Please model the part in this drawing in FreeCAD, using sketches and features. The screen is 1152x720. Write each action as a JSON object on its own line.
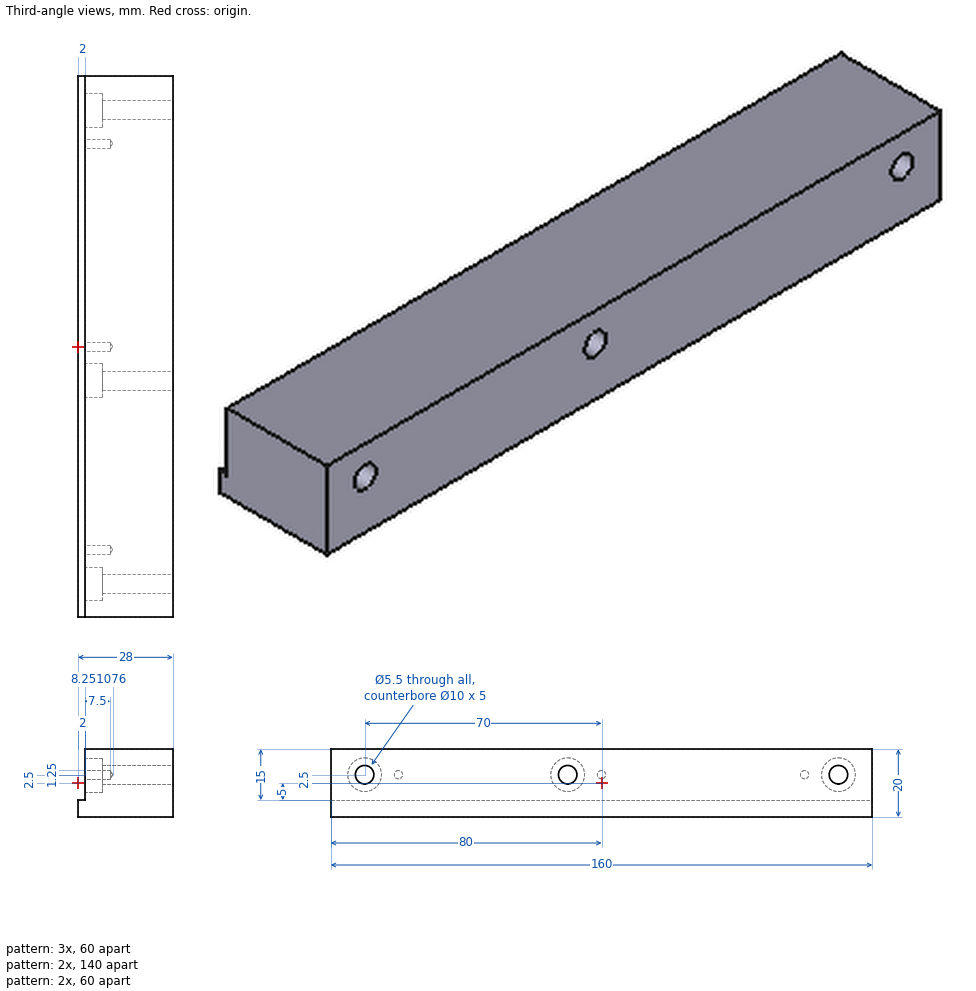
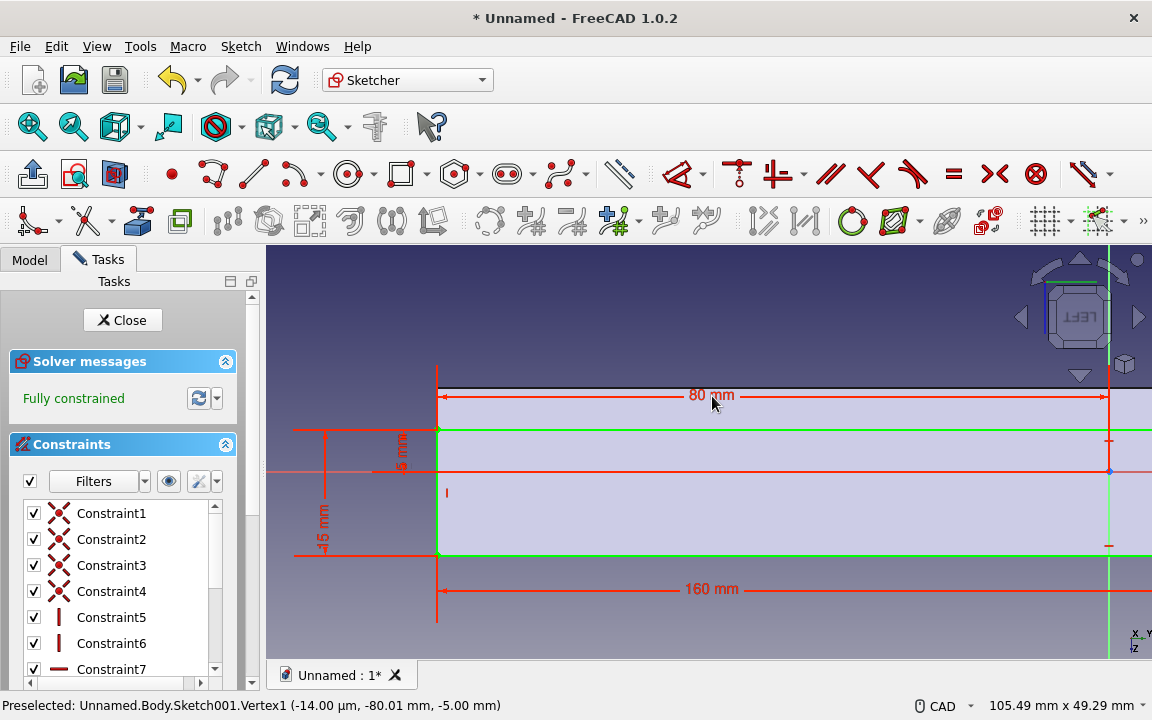
{"action": "left_click", "coordinate": [123, 320]}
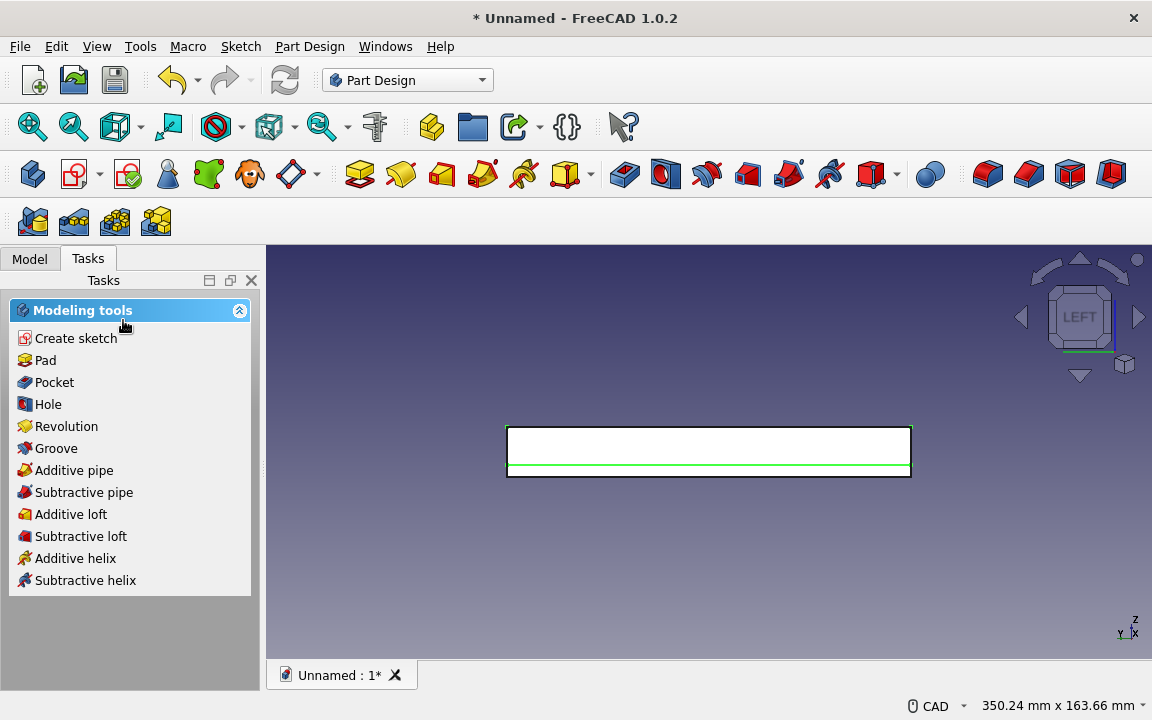
{"action": "left_click", "coordinate": [625, 174]}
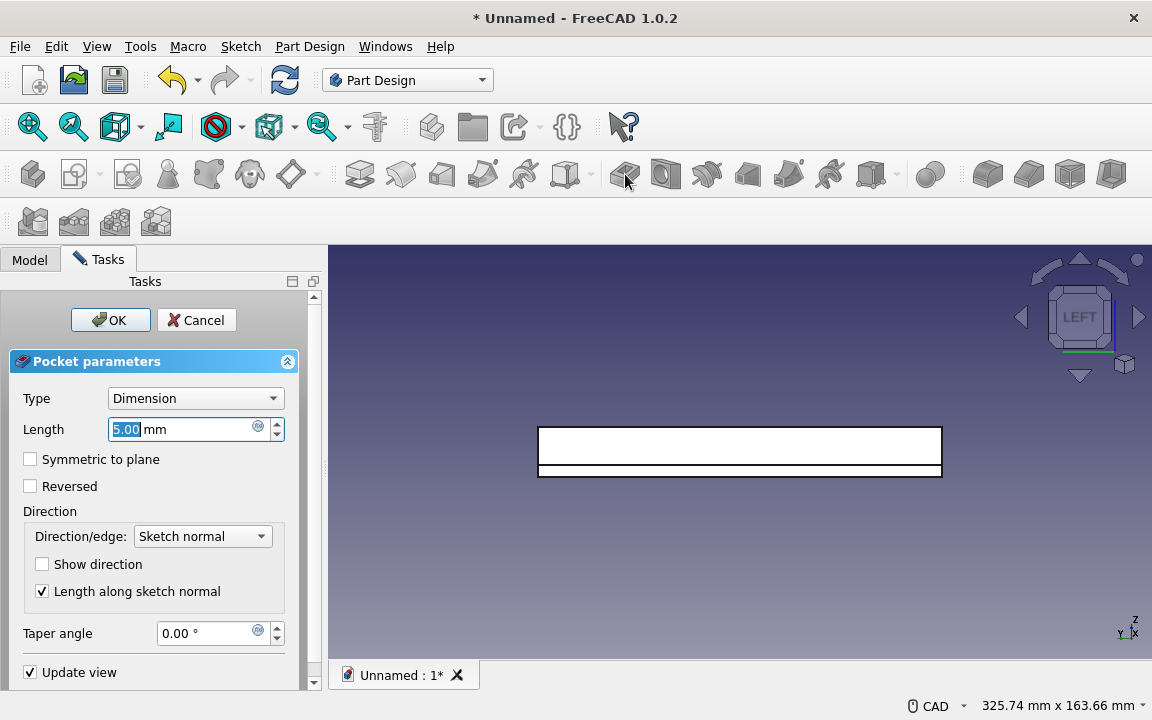
{"action": "type", "text": "2"}
{"action": "key", "text": "Tab"}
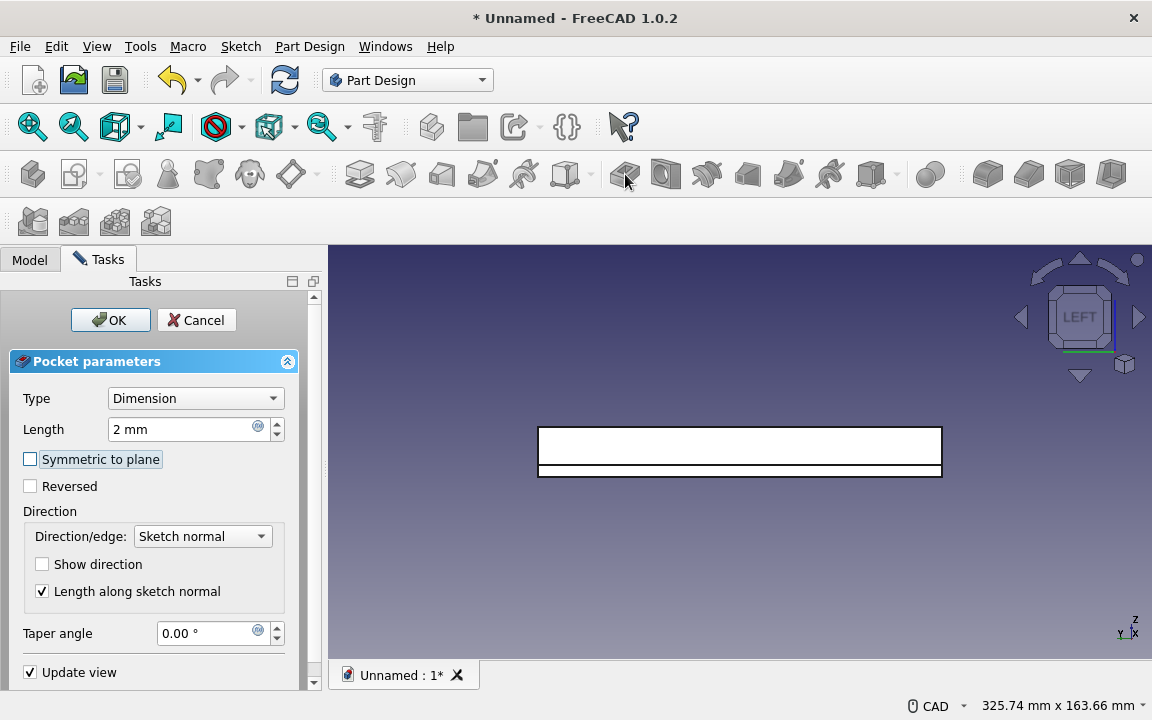
{"action": "left_click", "coordinate": [111, 320]}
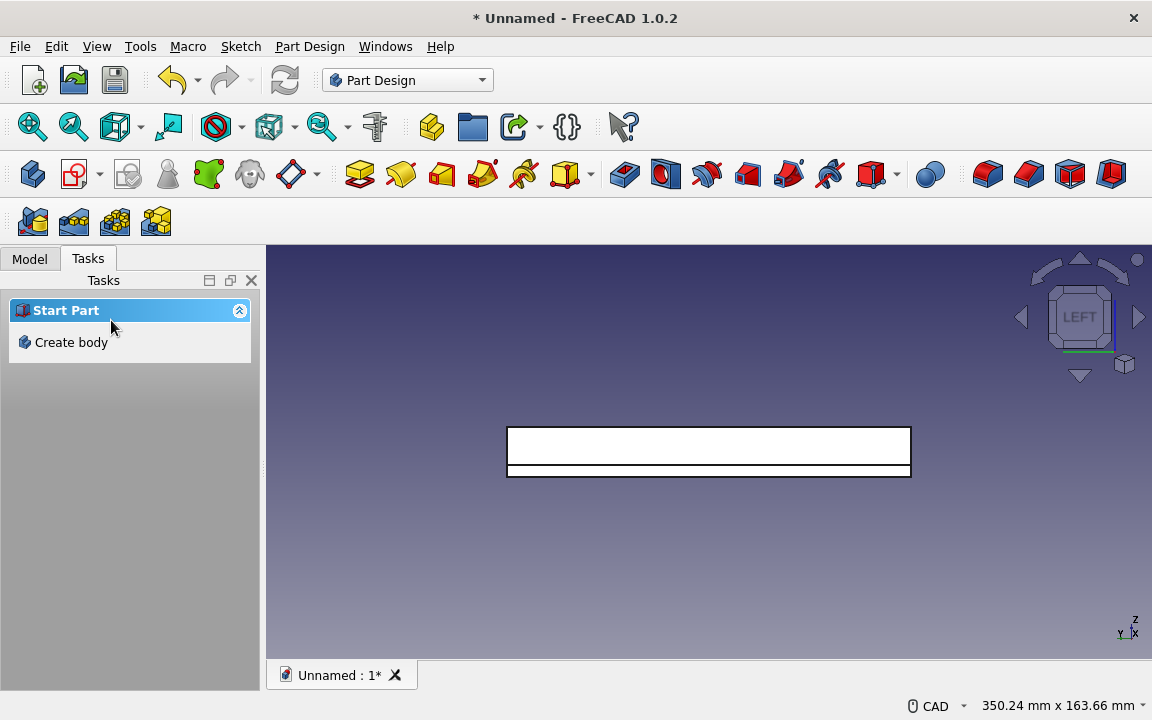
{"action": "left_click", "coordinate": [30, 258]}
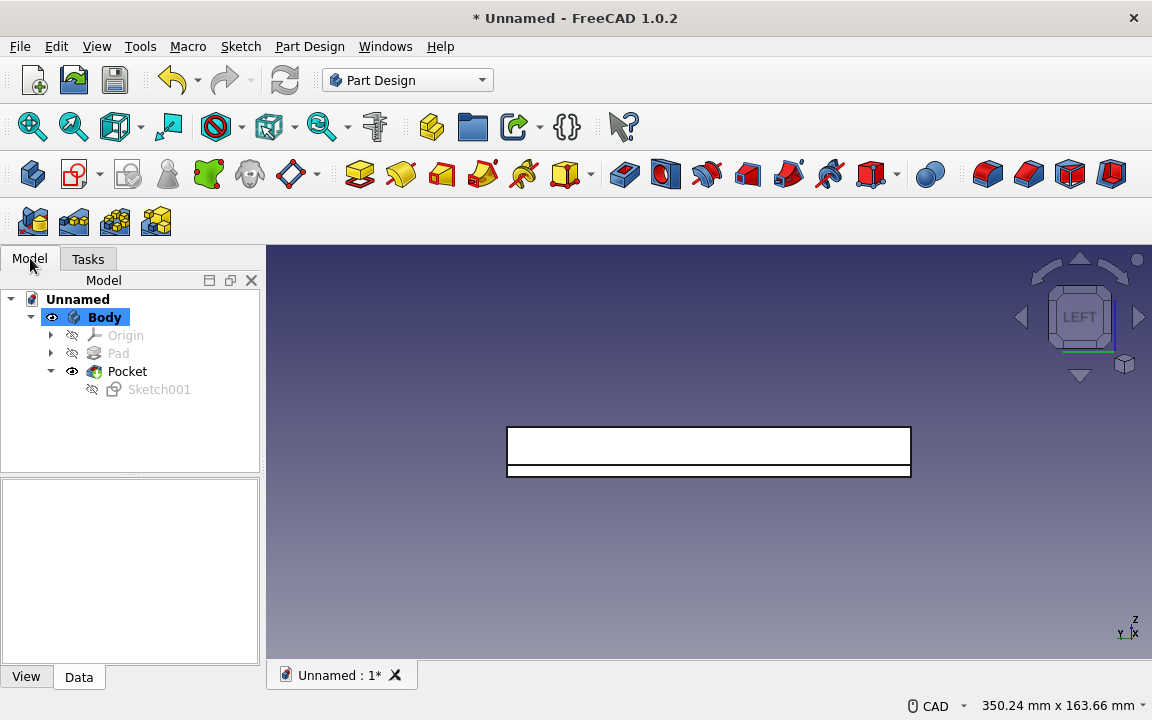
{"action": "left_click", "coordinate": [51, 335]}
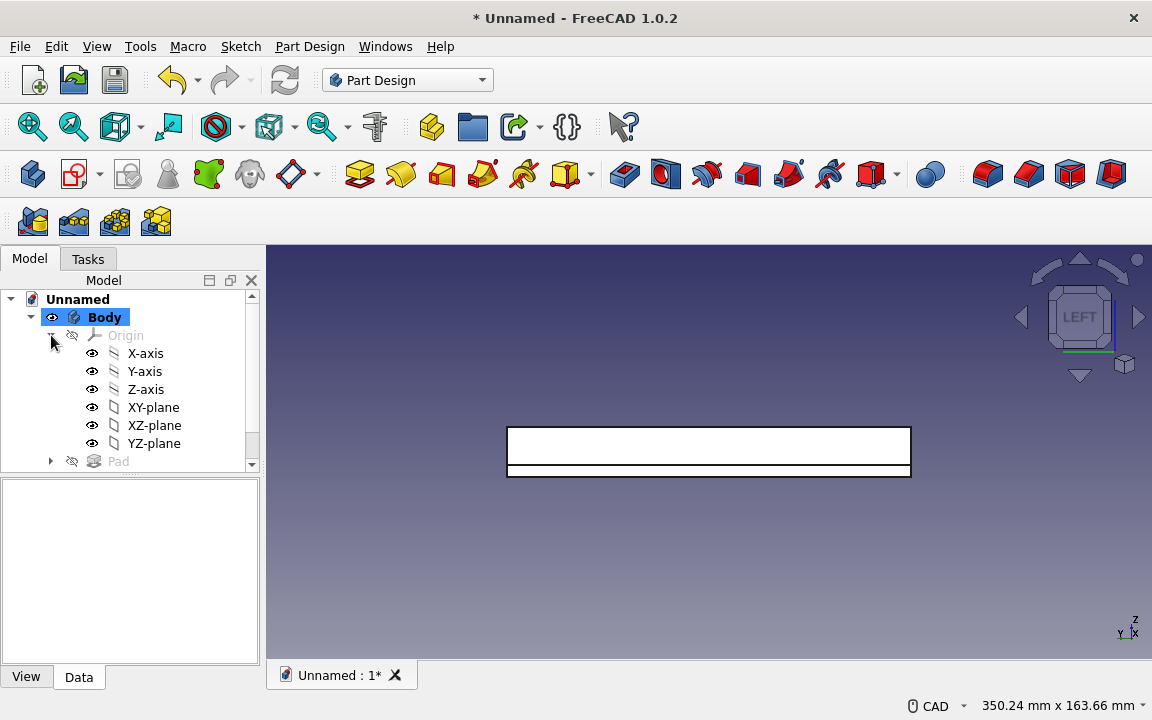
{"action": "left_click", "coordinate": [137, 425]}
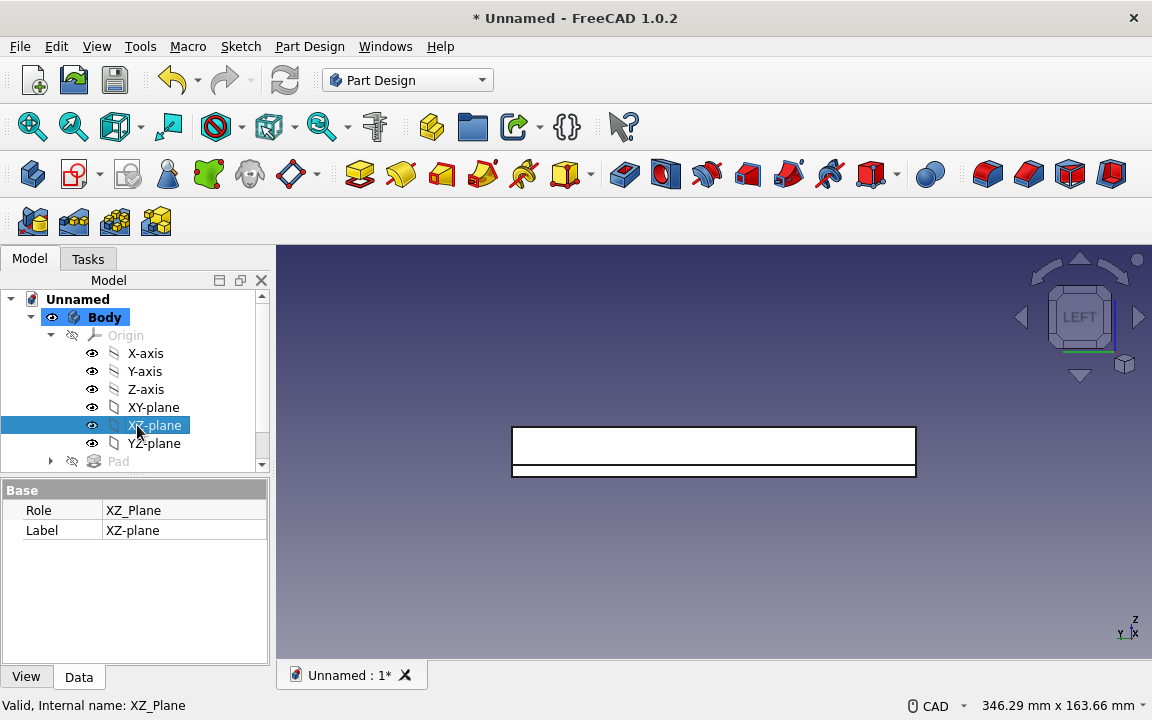
{"action": "left_click", "coordinate": [290, 174]}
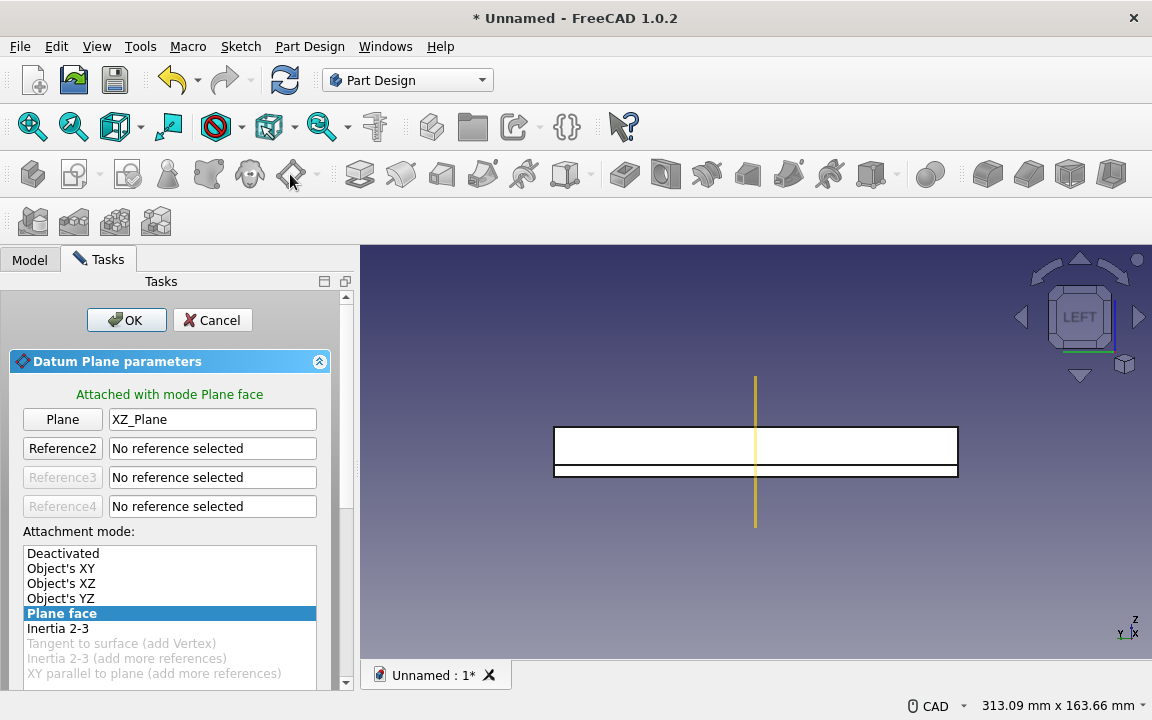
{"action": "scroll", "coordinate": [346, 490], "scroll_direction": "down", "scroll_amount": 4}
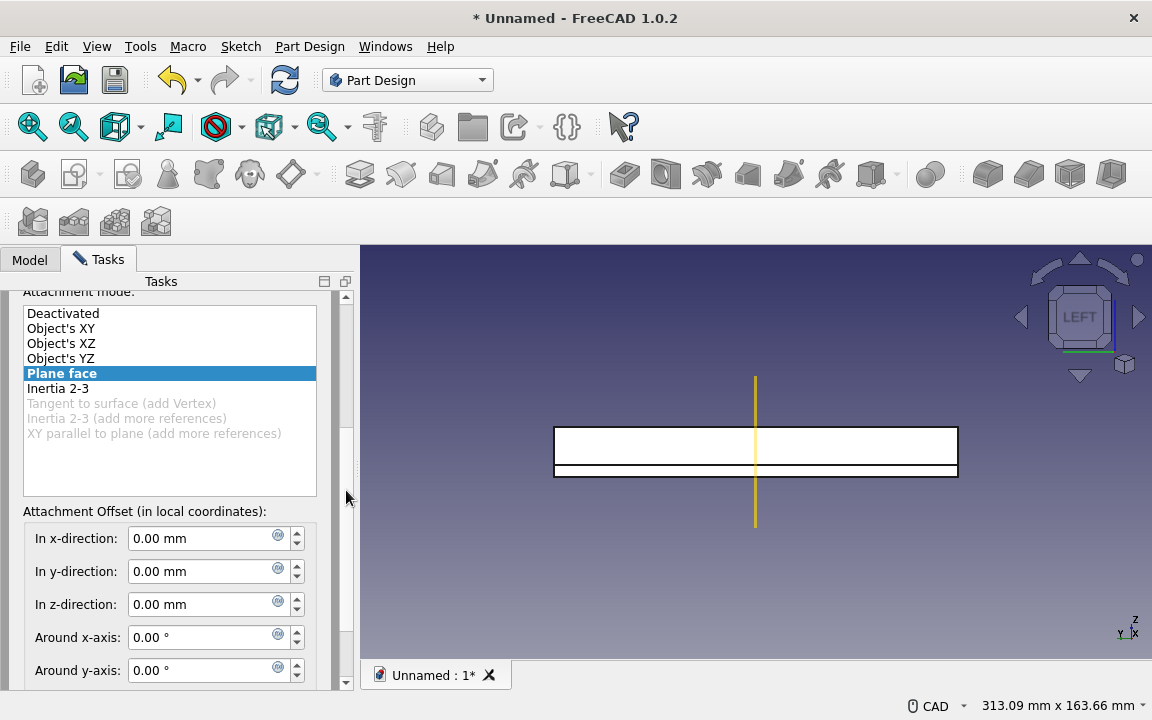
{"action": "triple_click", "coordinate": [210, 604]}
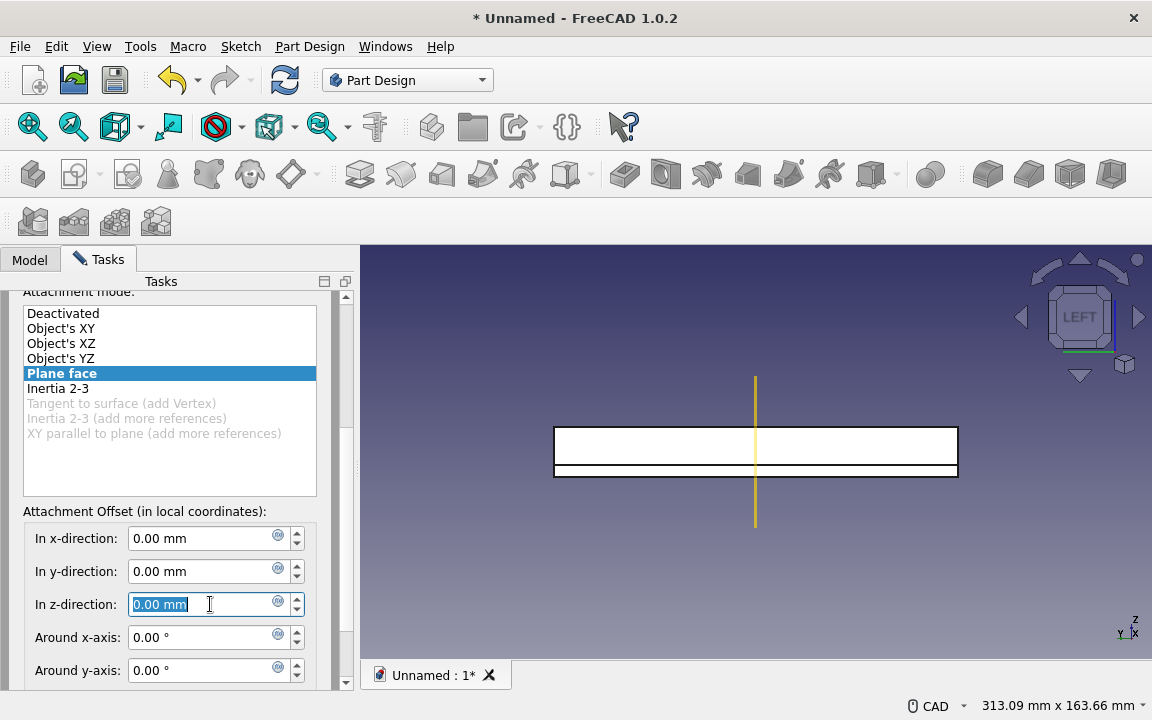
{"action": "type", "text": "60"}
{"action": "key", "text": "Tab"}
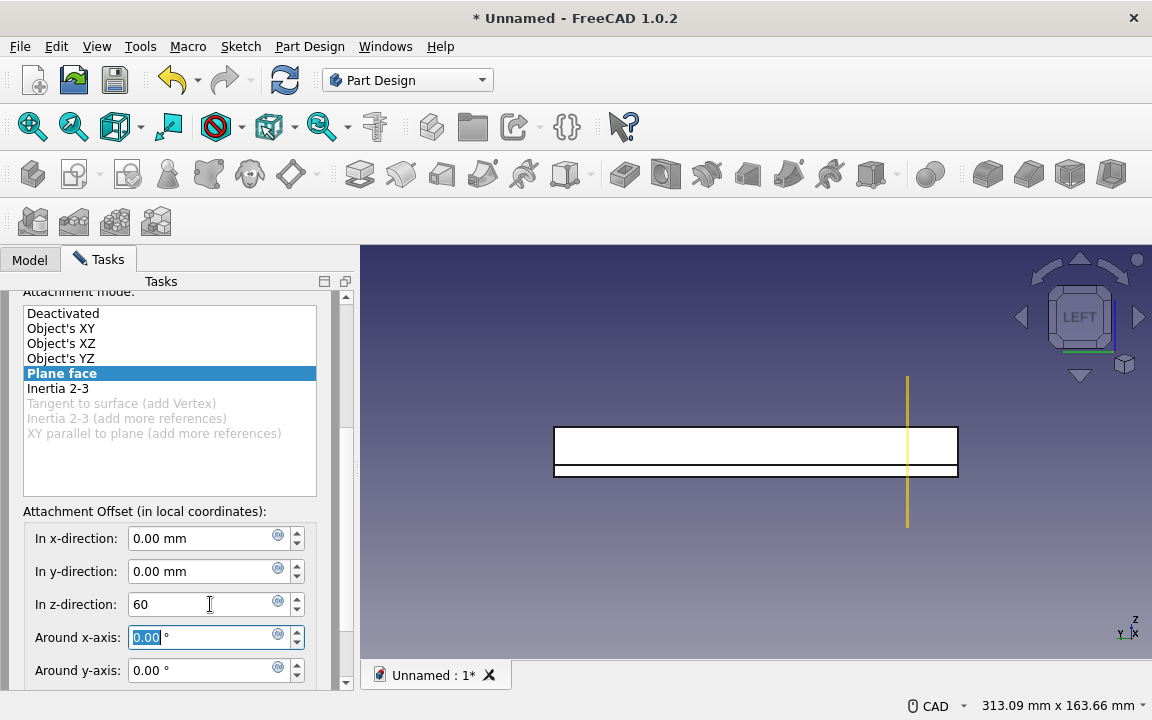
{"action": "scroll", "coordinate": [346, 490], "scroll_direction": "up", "scroll_amount": 5}